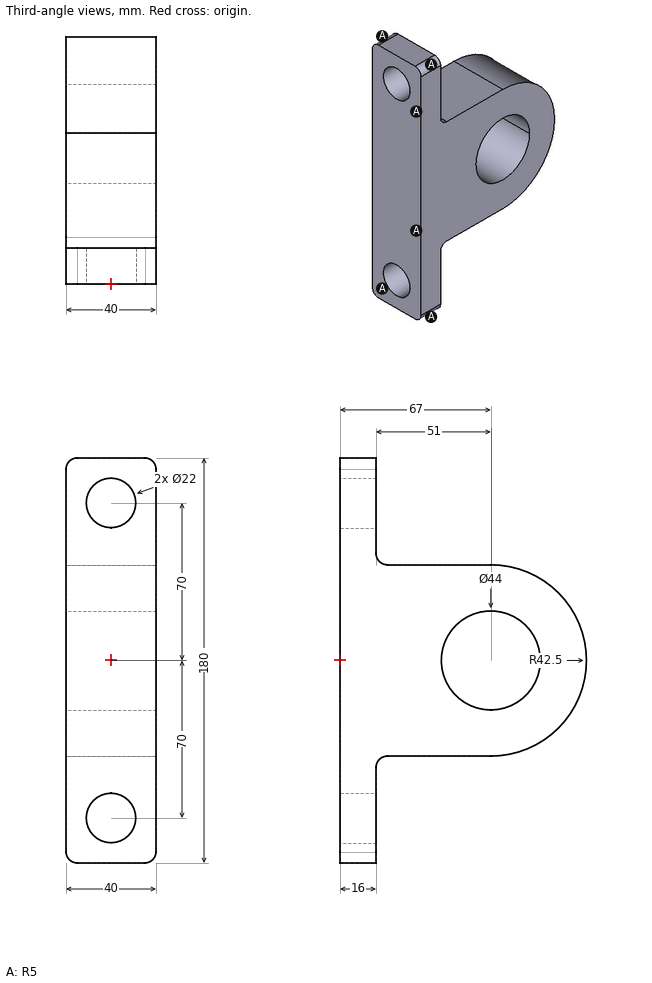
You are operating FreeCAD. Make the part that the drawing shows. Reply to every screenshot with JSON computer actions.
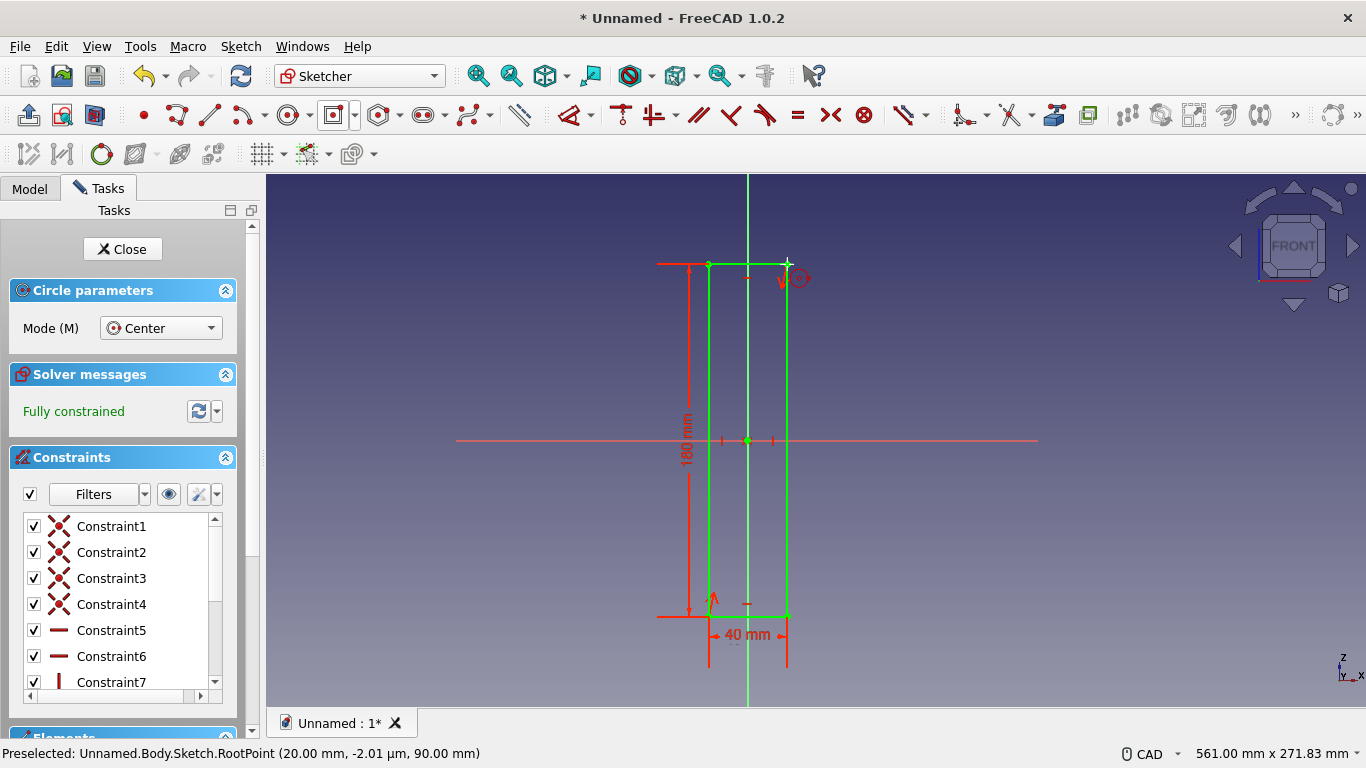
{"action": "left_click", "coordinate": [748, 303]}
{"action": "mouse_move", "coordinate": [763, 288]}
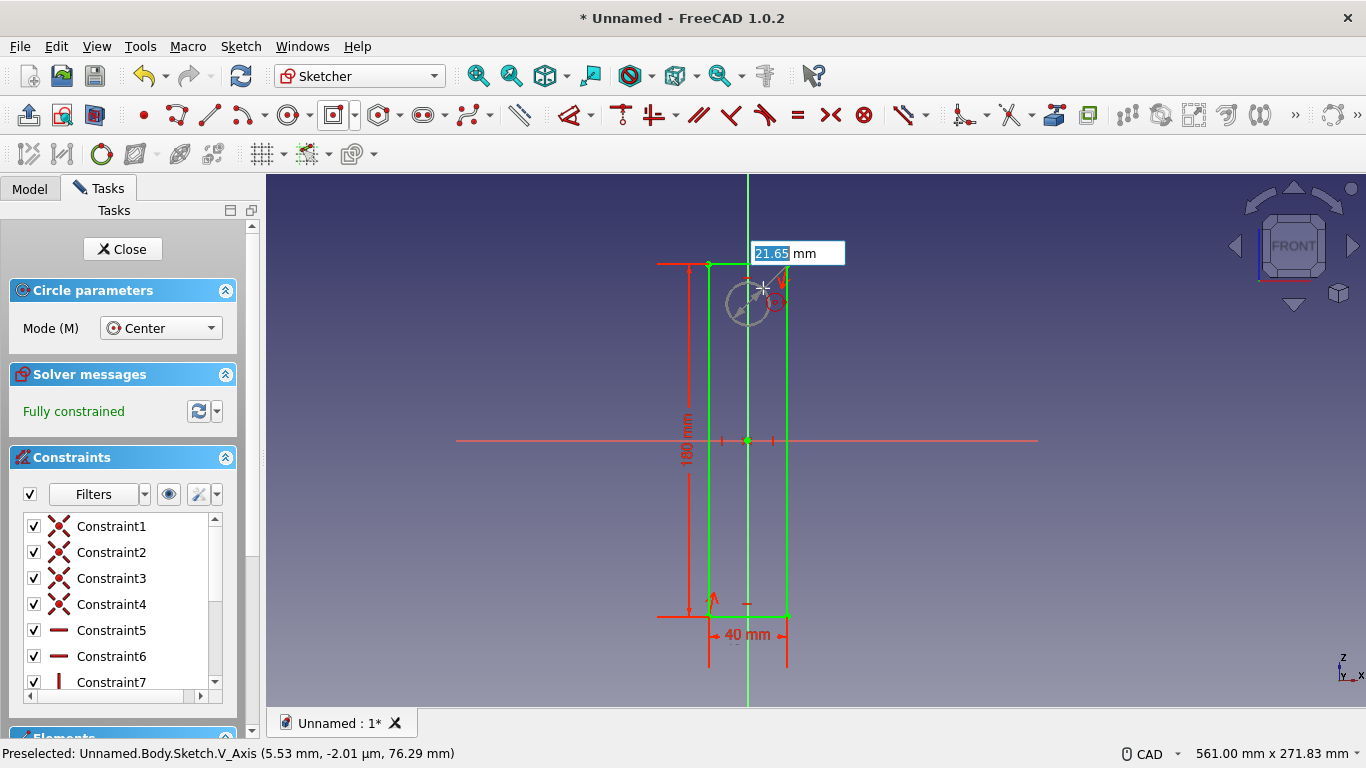
{"action": "type", "text": "22"}
{"action": "key", "text": "Return"}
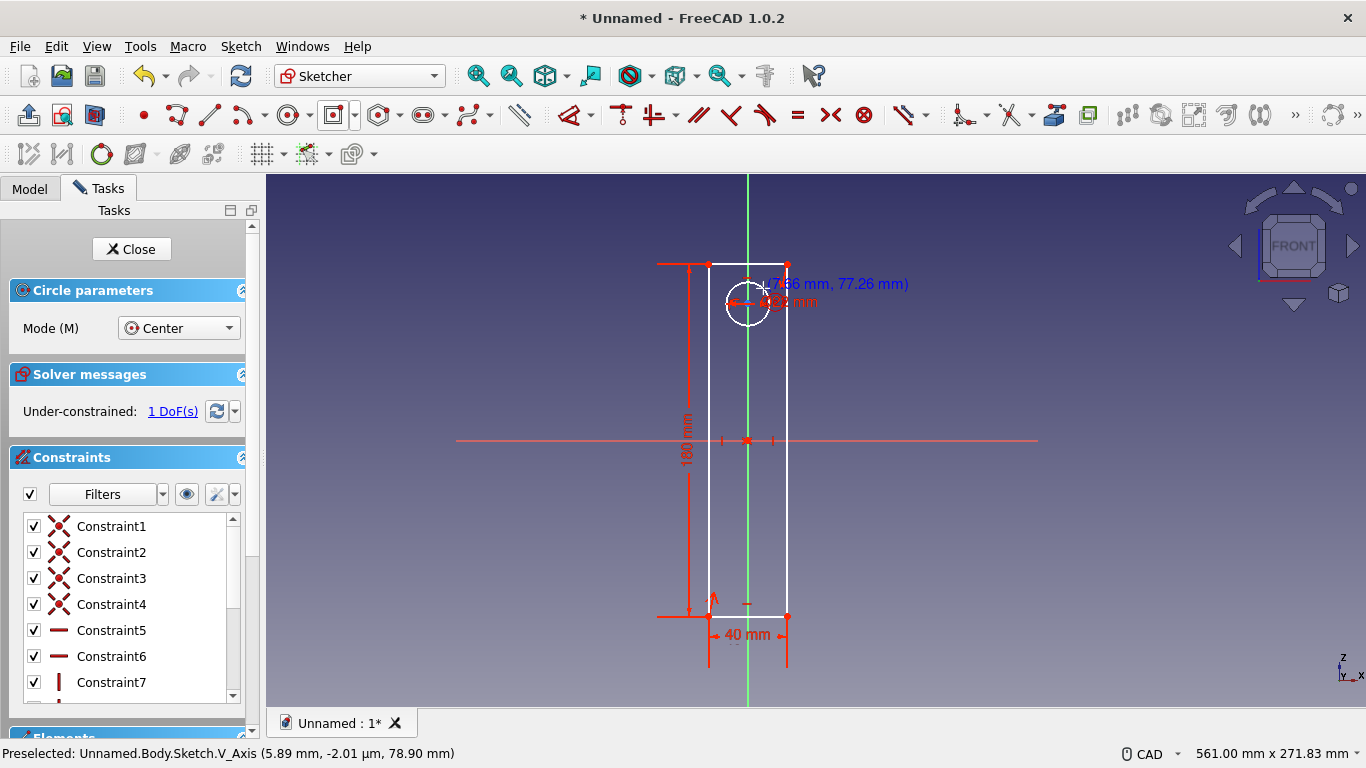
{"action": "left_click", "coordinate": [748, 578]}
{"action": "mouse_move", "coordinate": [763, 563]}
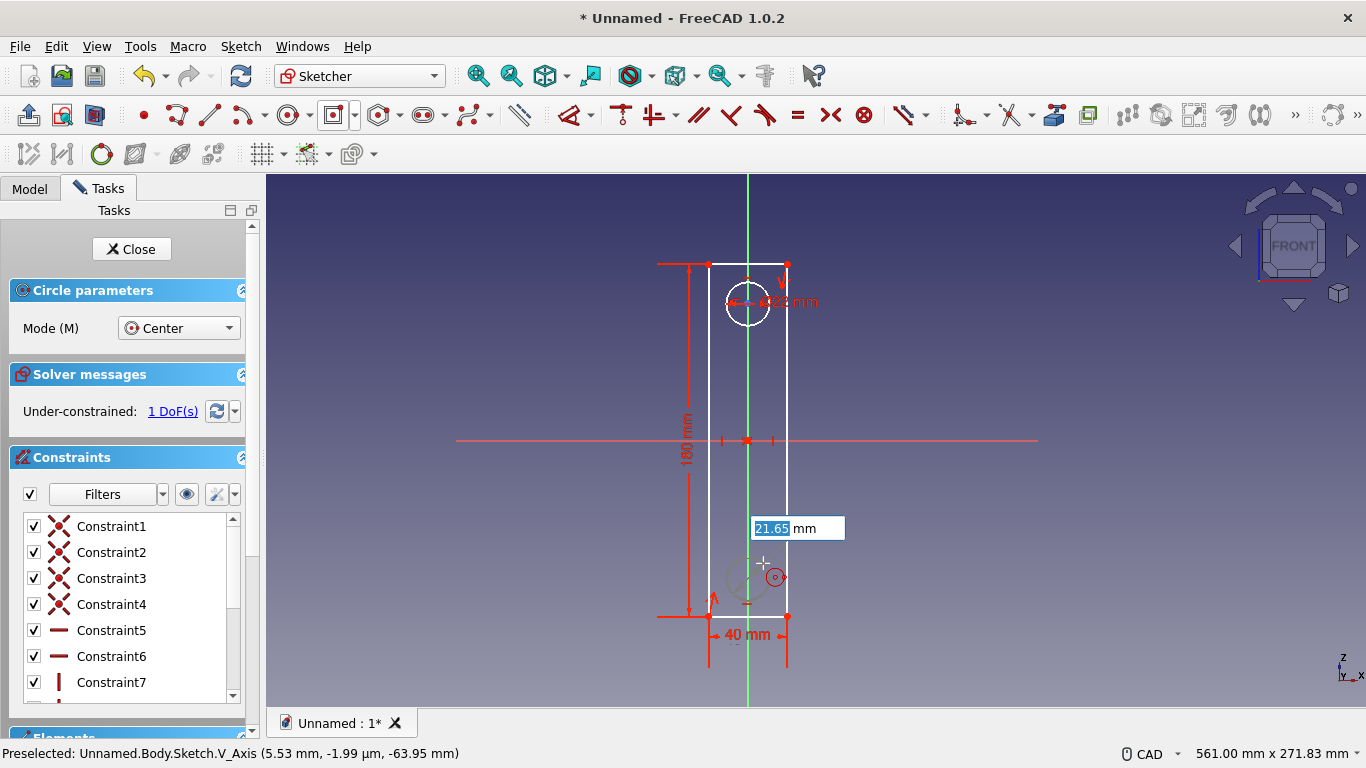
{"action": "type", "text": "22"}
{"action": "key", "text": "Return"}
{"action": "key", "text": "Escape"}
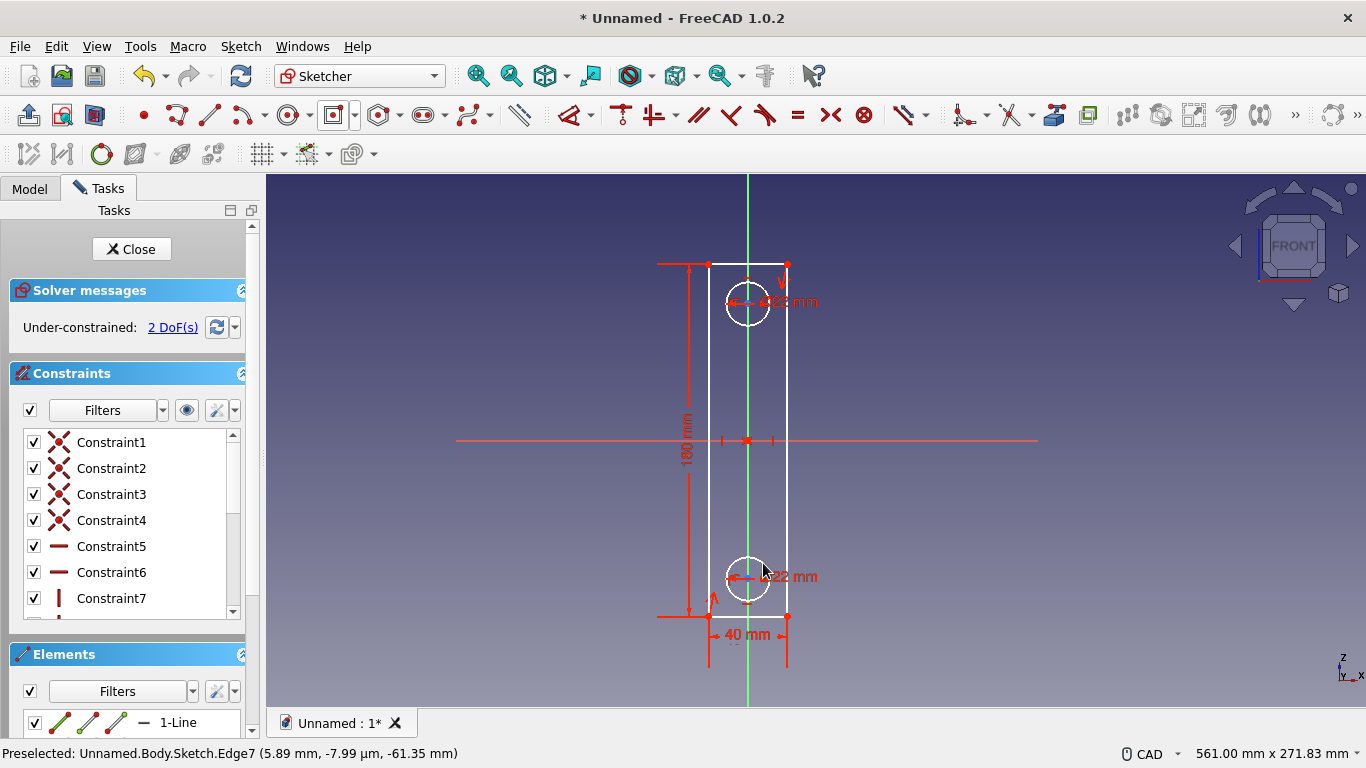
{"action": "left_click", "coordinate": [748, 304]}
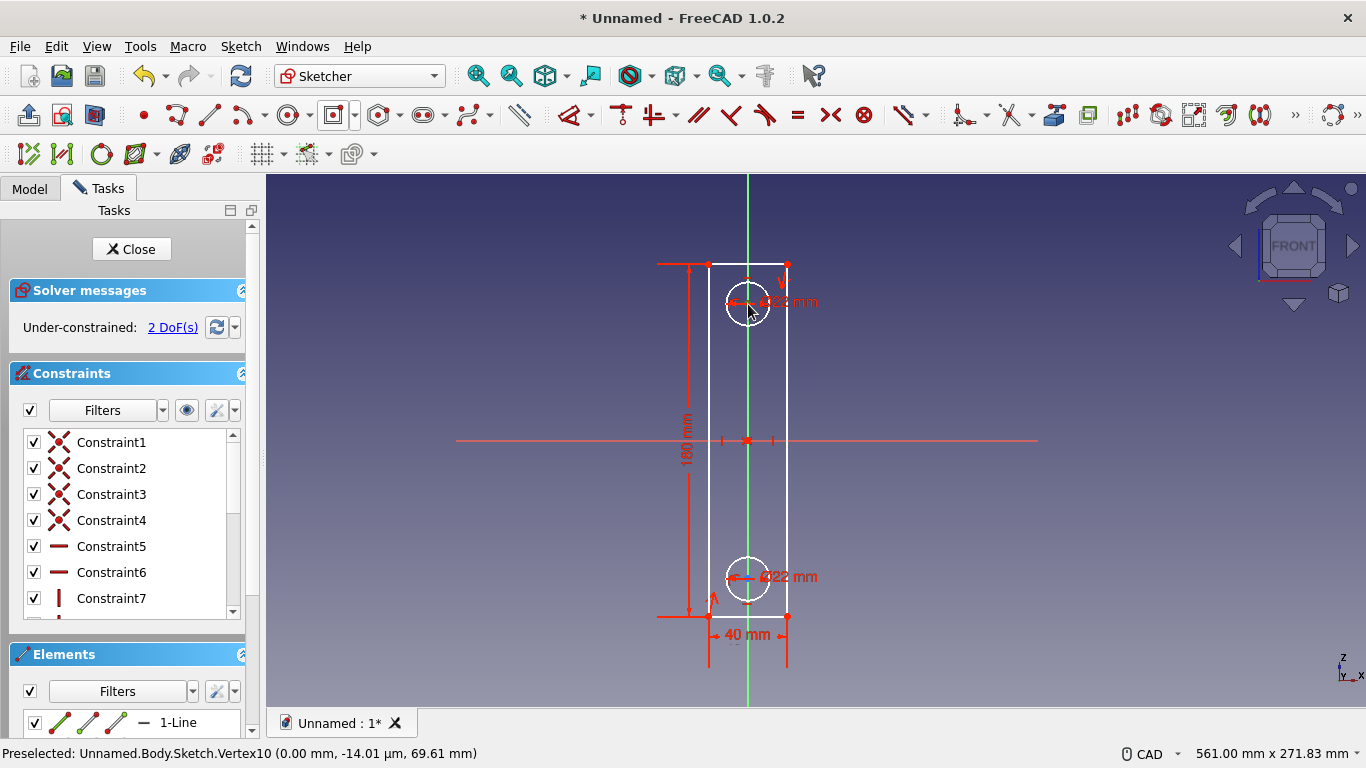
{"action": "left_click", "coordinate": [590, 116]}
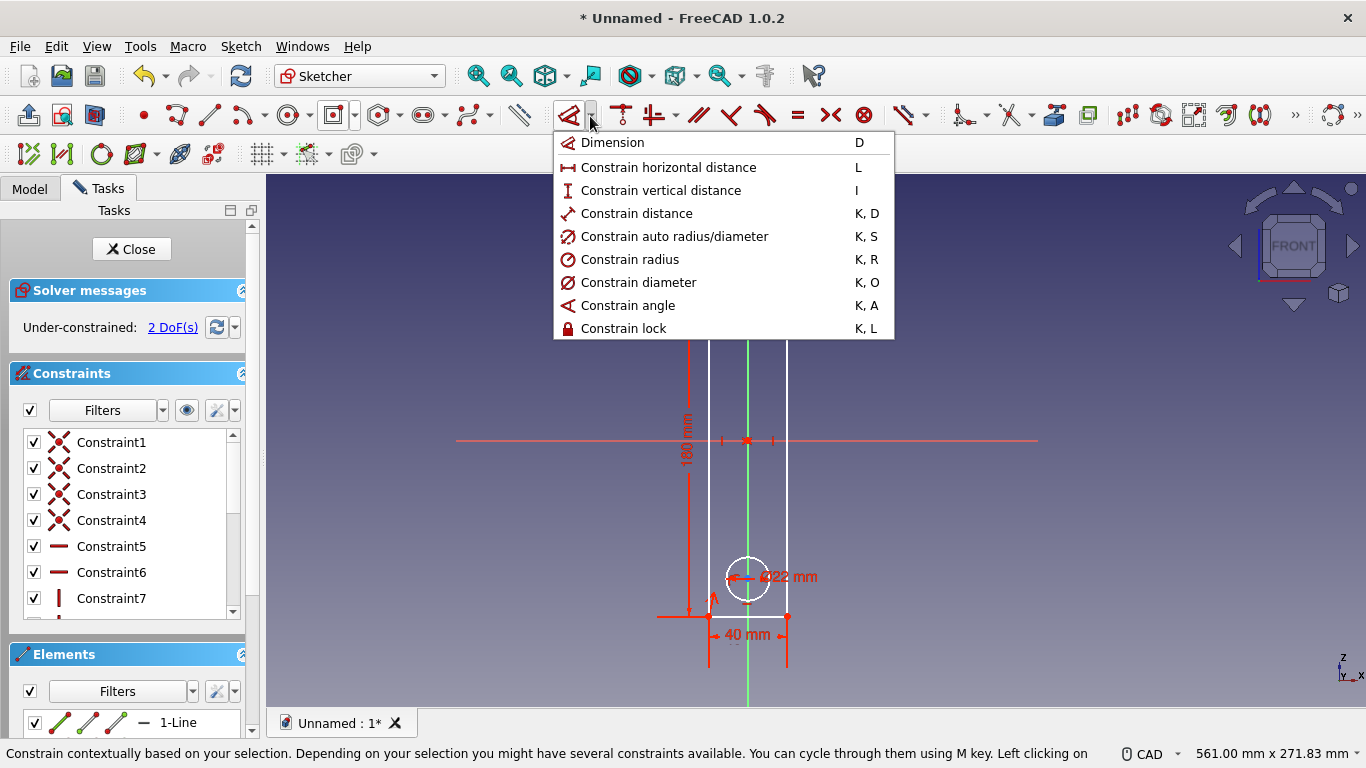
{"action": "left_click", "coordinate": [724, 190]}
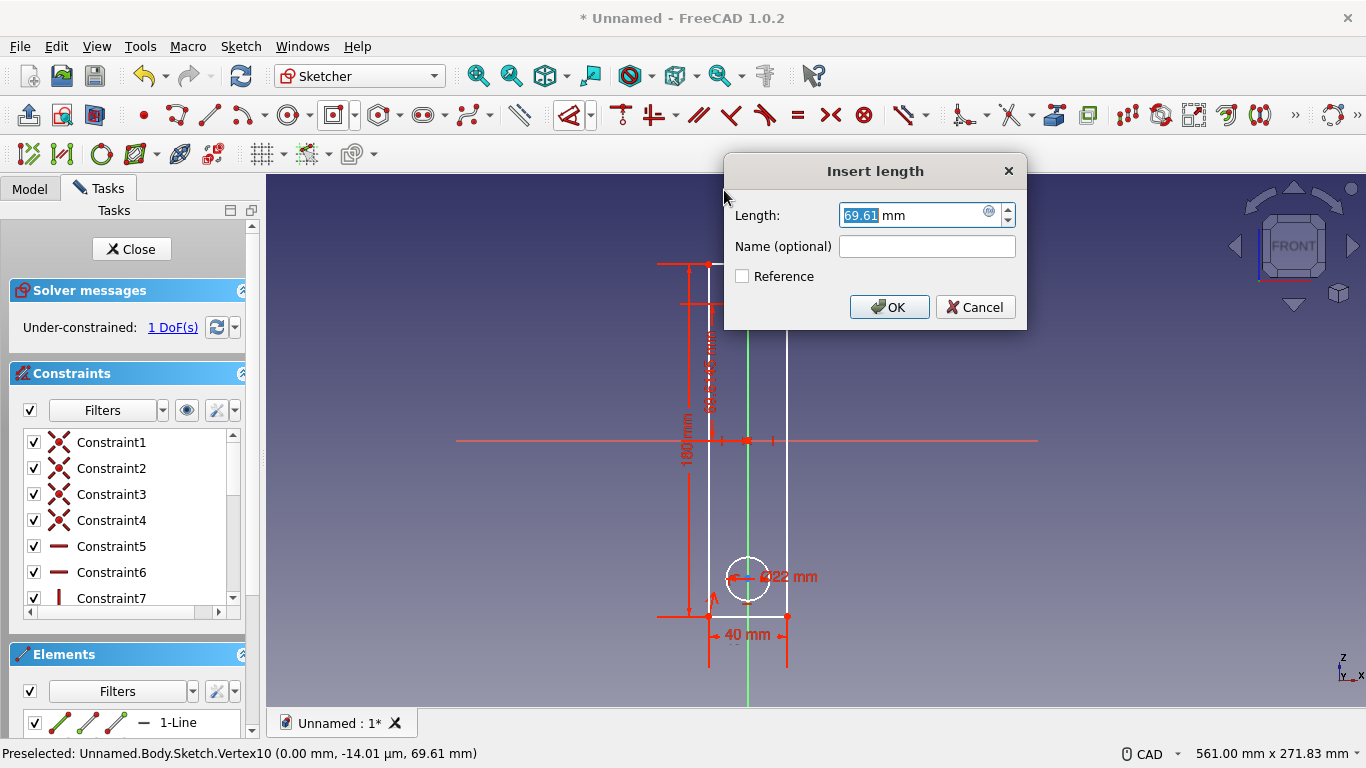
{"action": "type", "text": "70"}
{"action": "key", "text": "Return"}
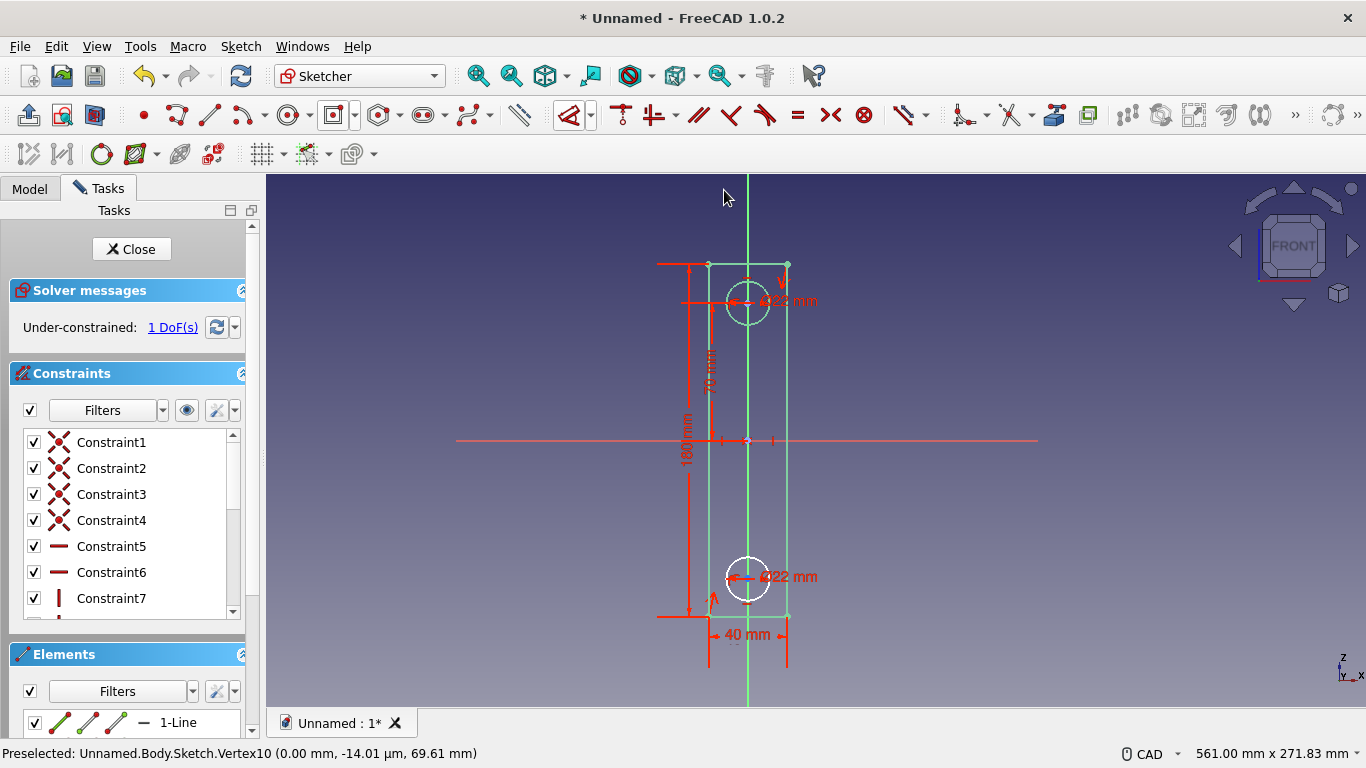
{"action": "left_click", "coordinate": [748, 579]}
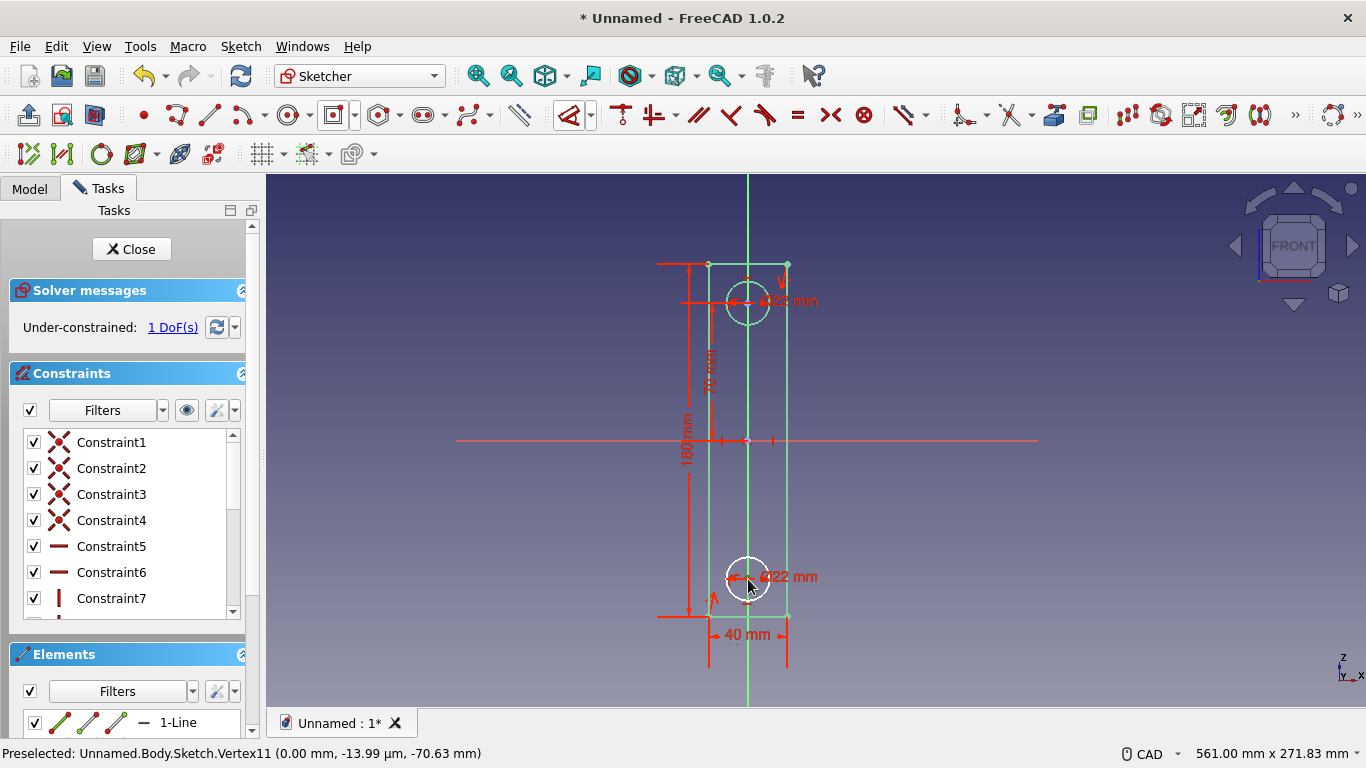
{"action": "key", "text": "i"}